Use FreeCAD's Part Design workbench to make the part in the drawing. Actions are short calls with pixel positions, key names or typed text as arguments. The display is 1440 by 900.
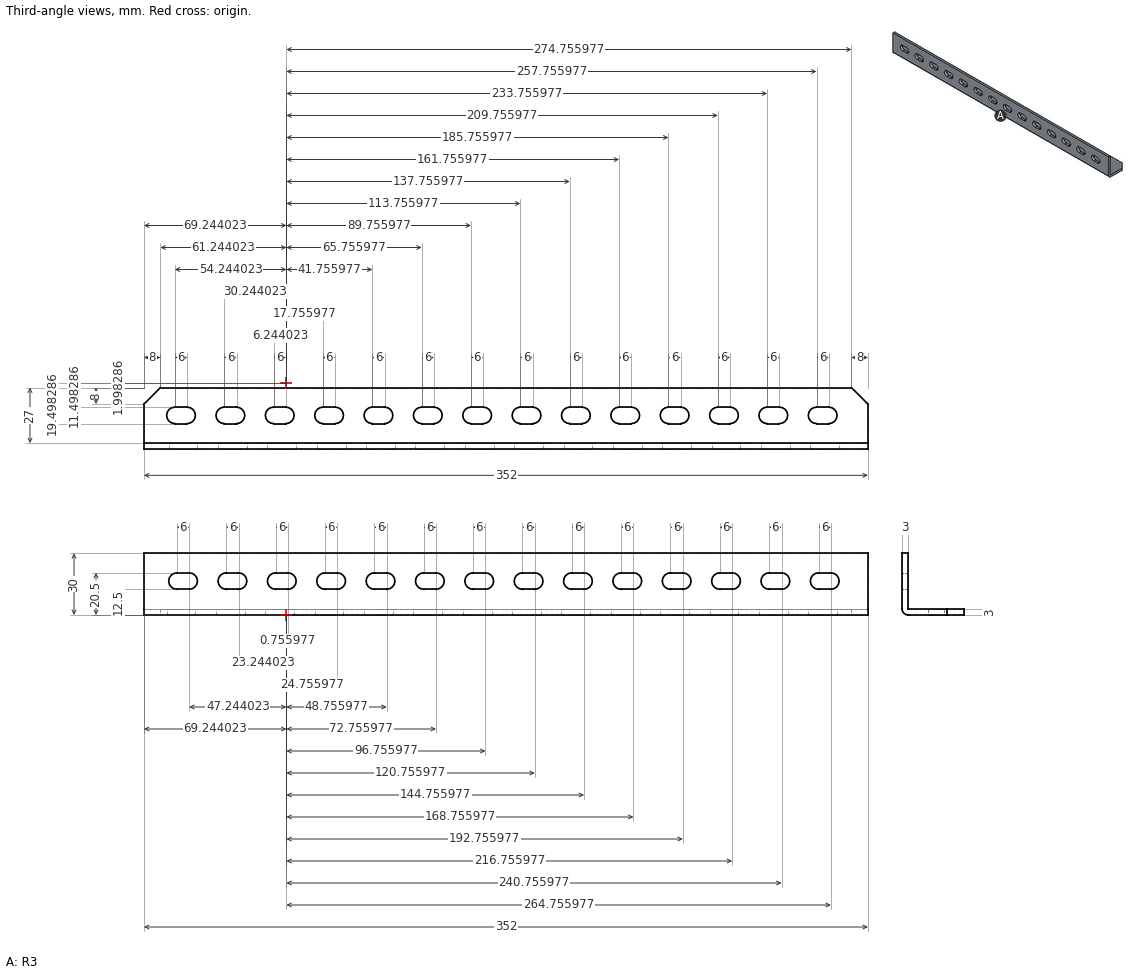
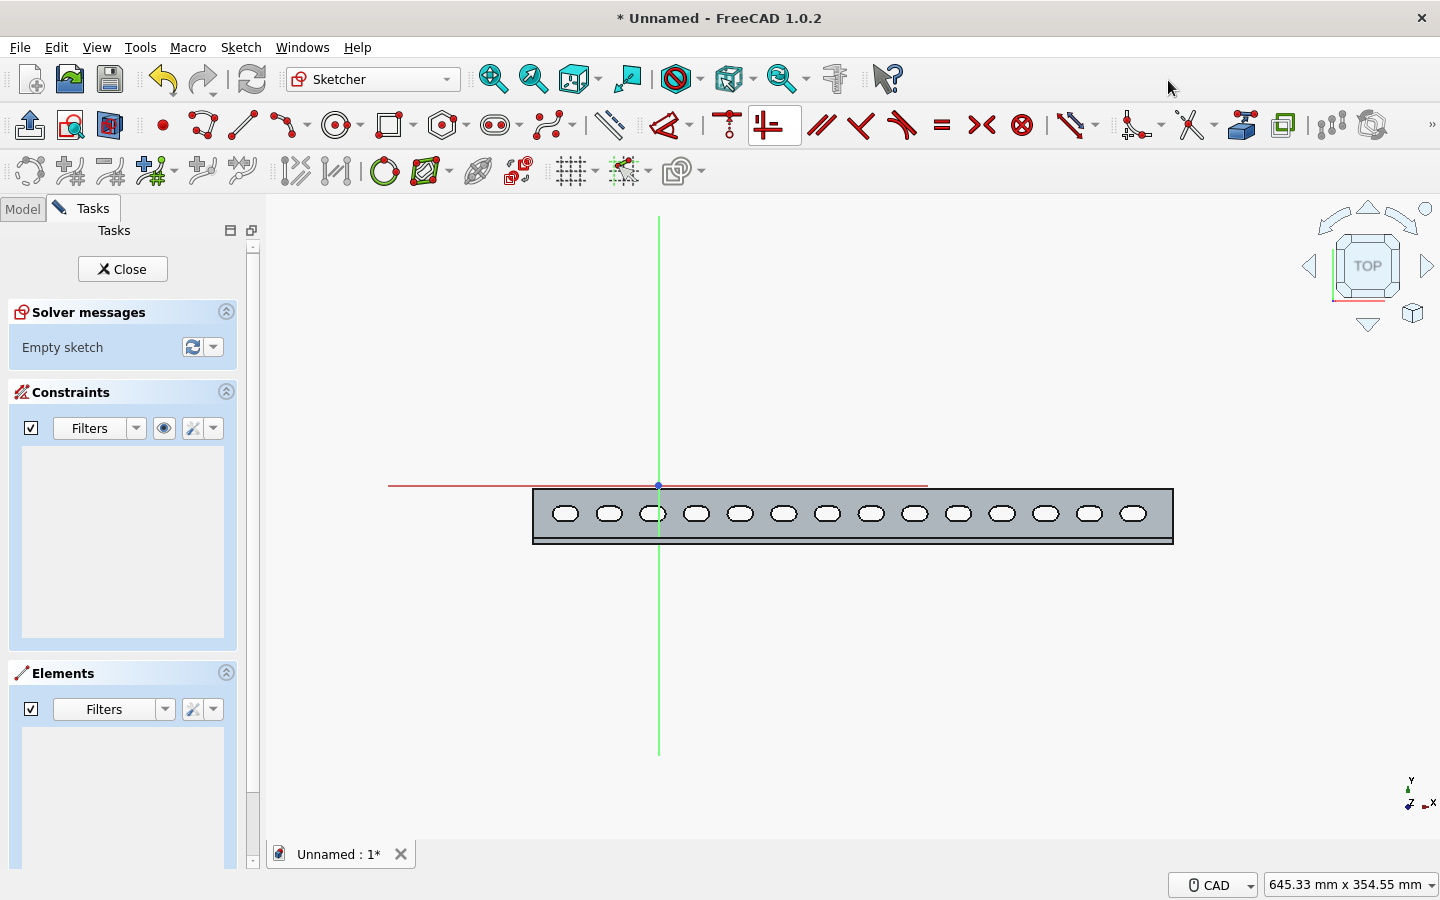
click(204, 126)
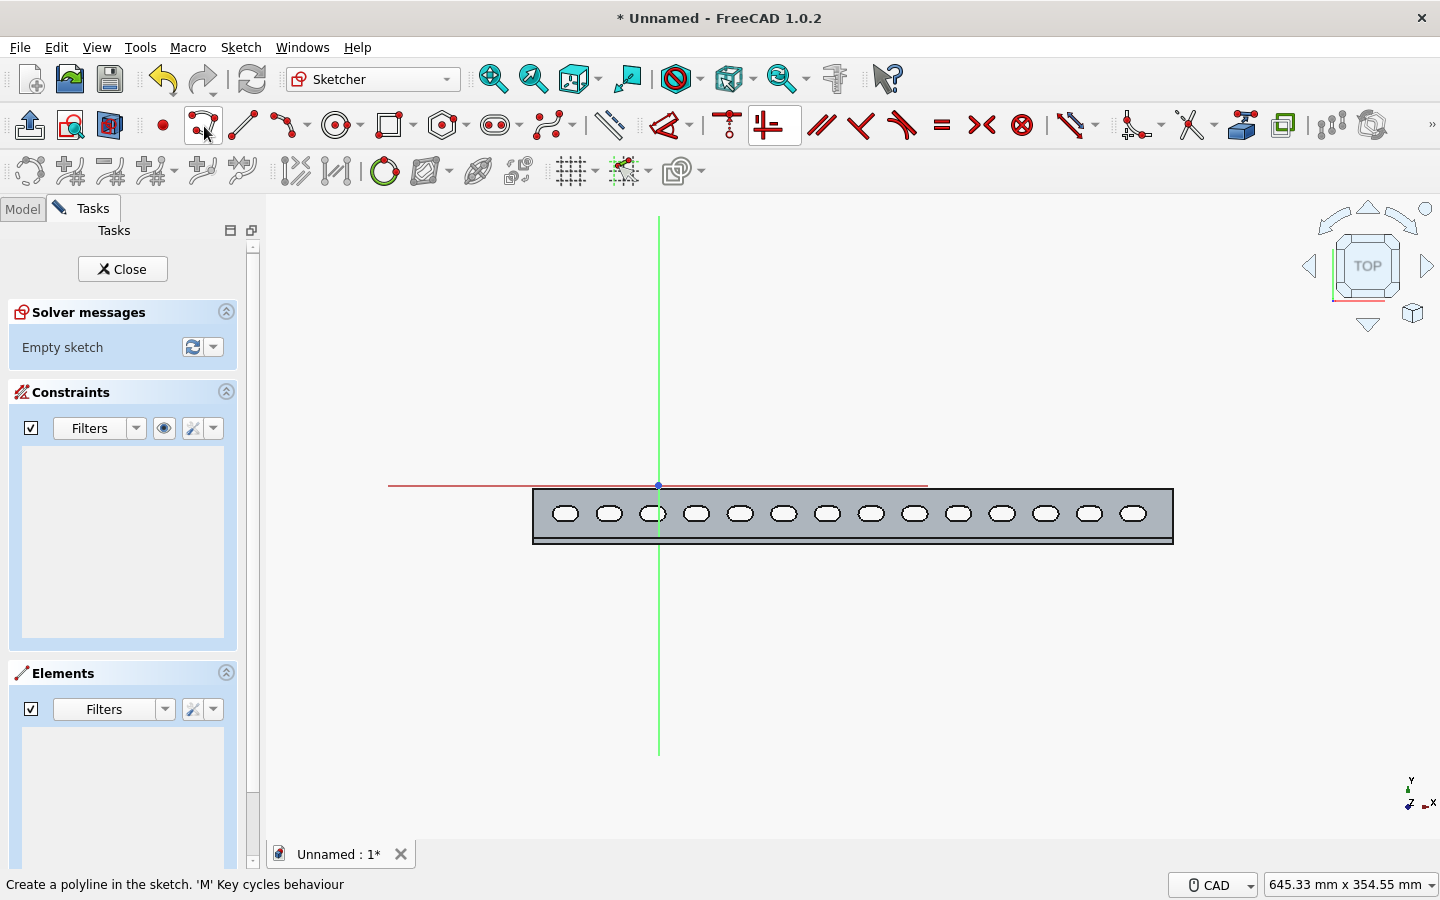
scroll(547, 489, up, 8)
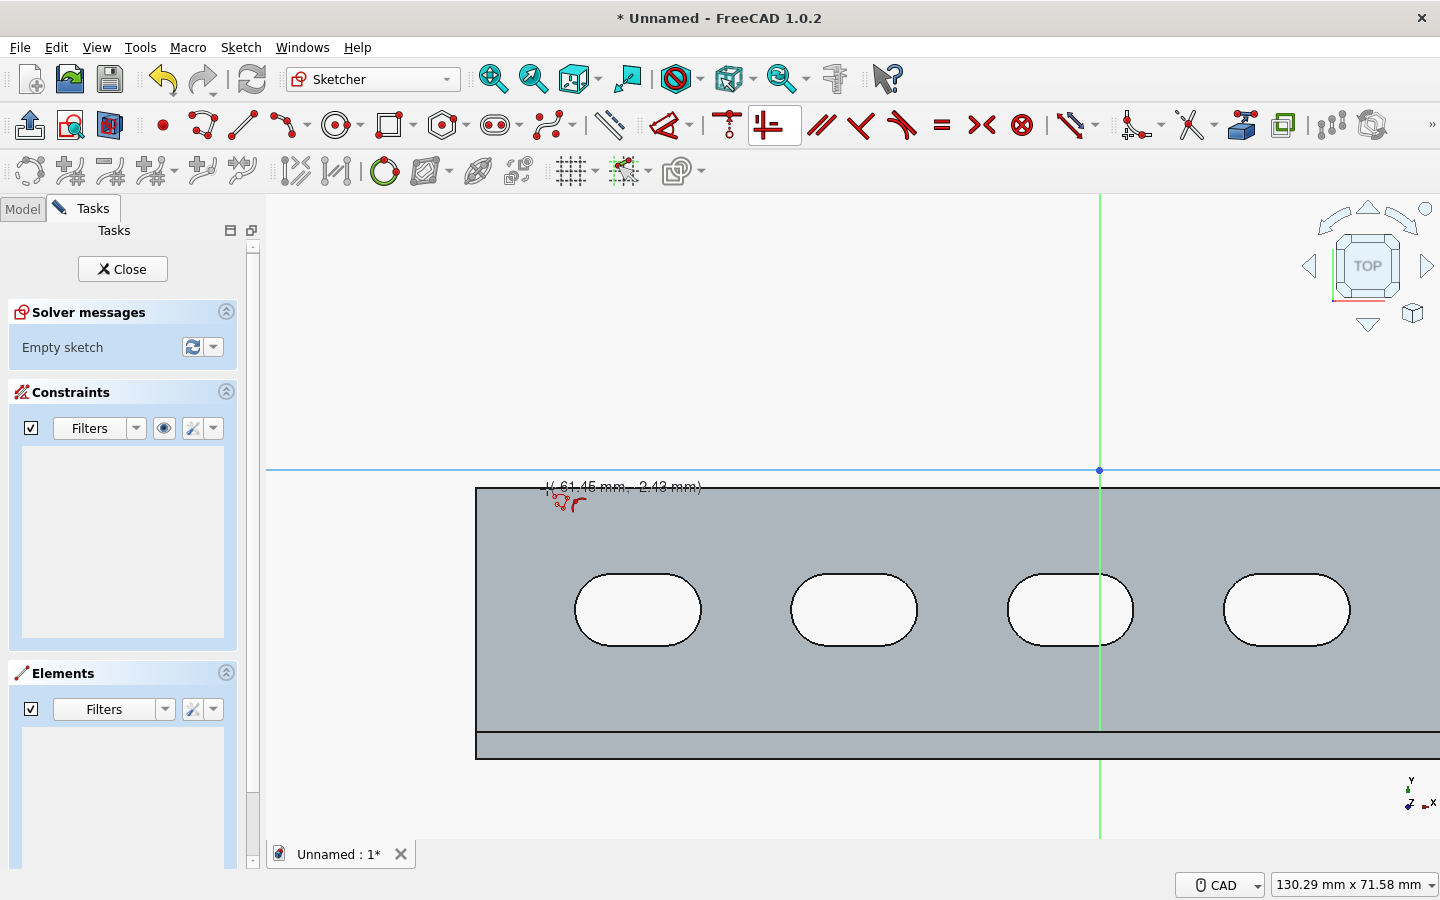
click(548, 488)
click(476, 488)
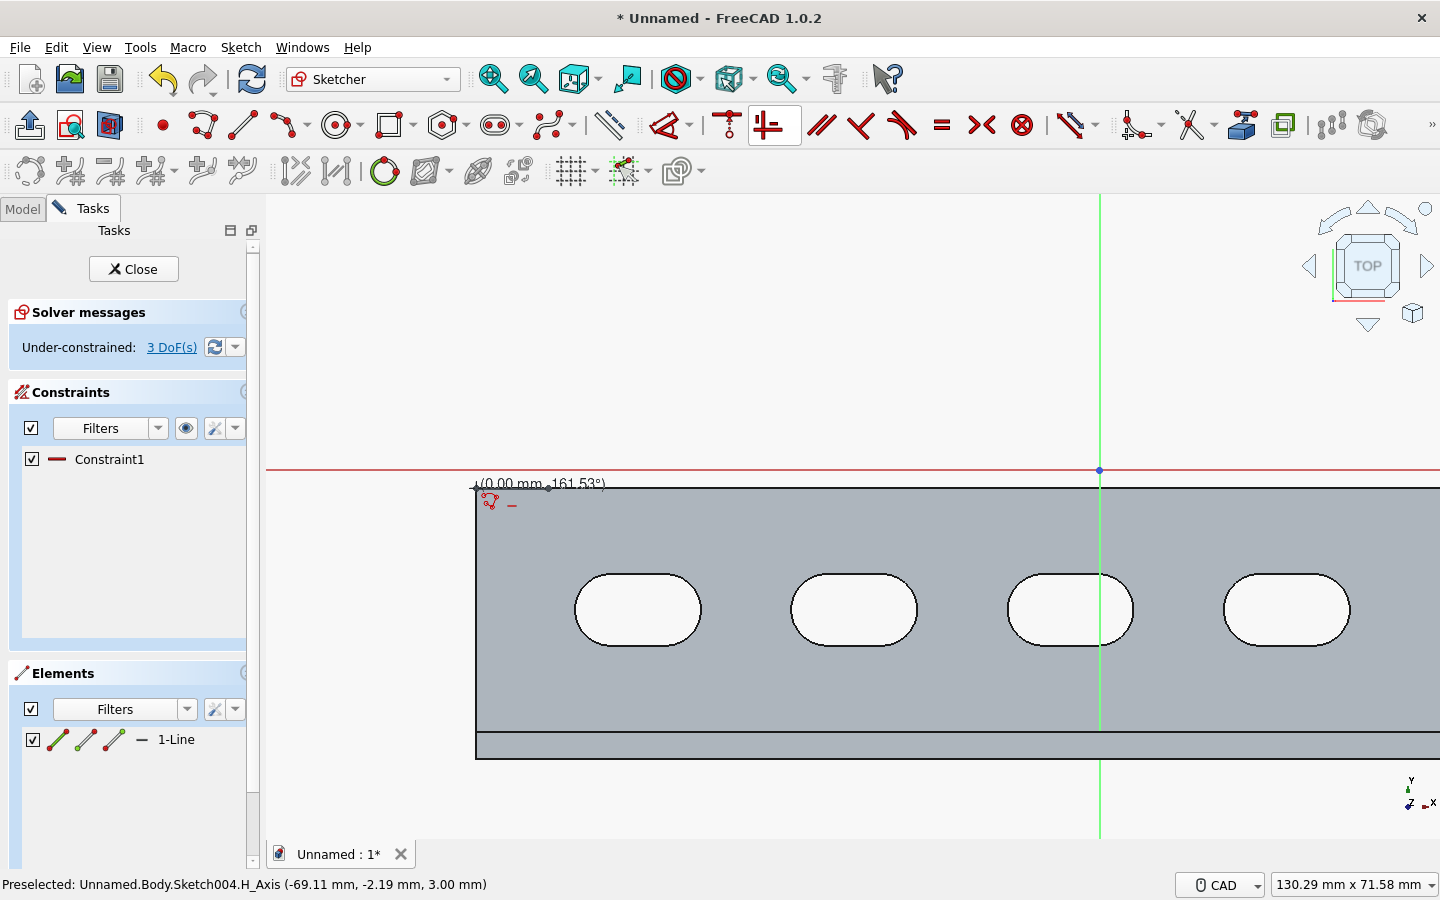
scroll(461, 517, down, 8)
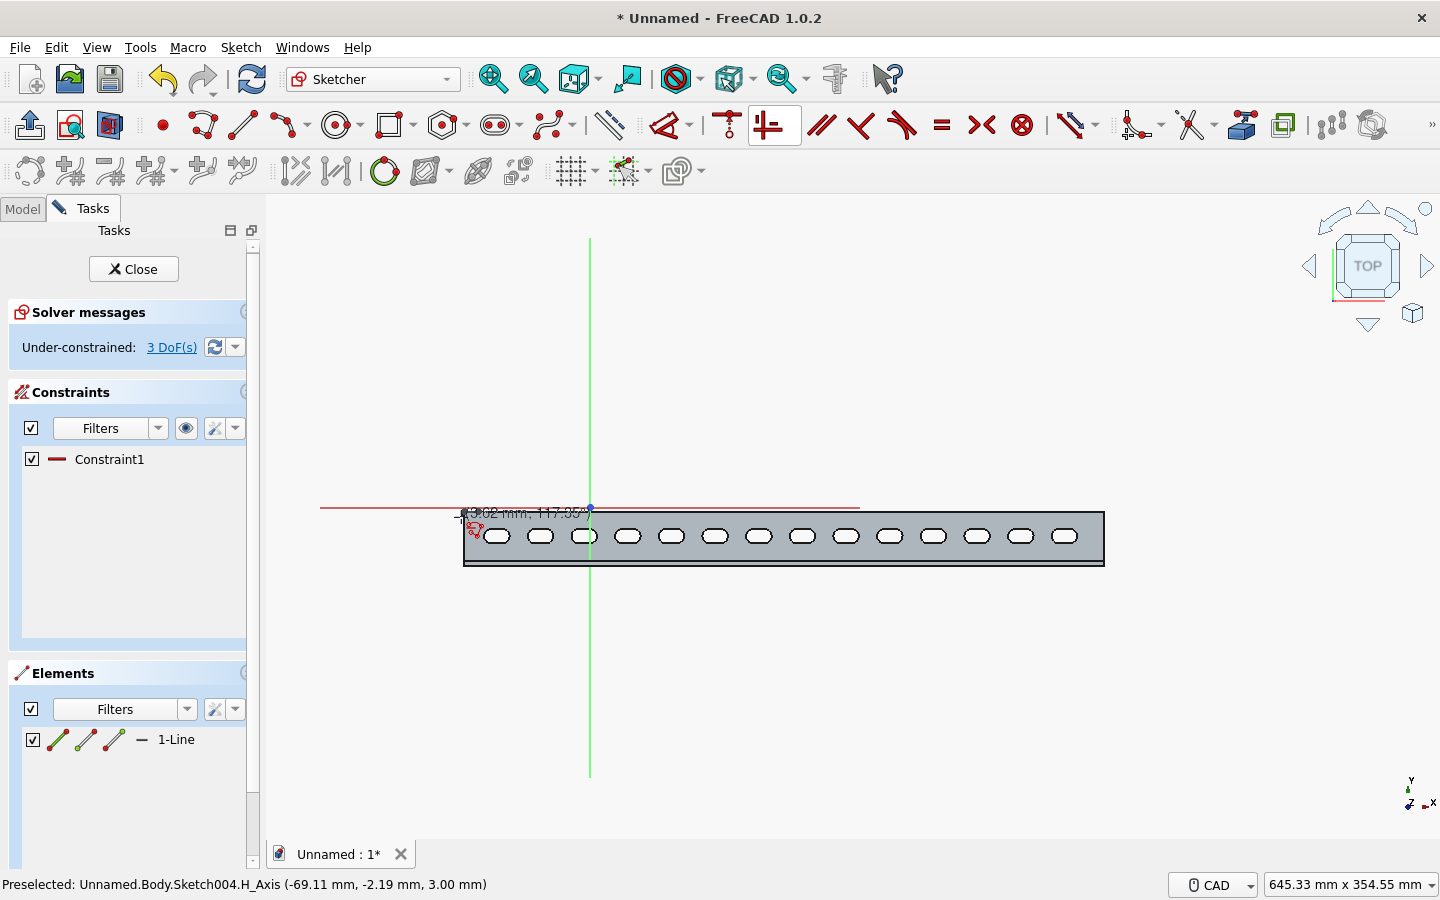
click(464, 526)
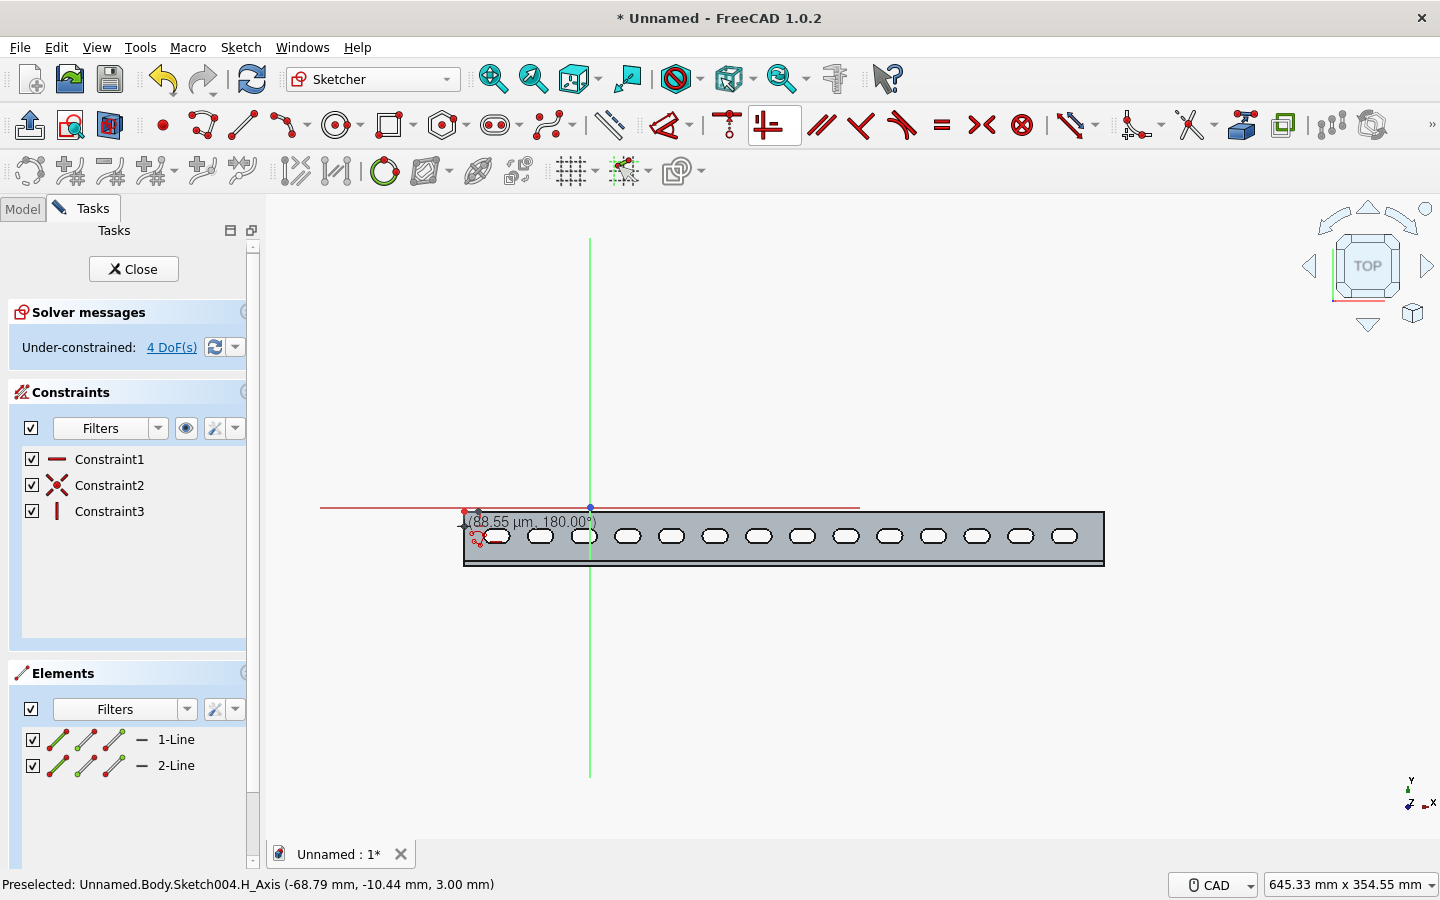
scroll(479, 512, up, 8)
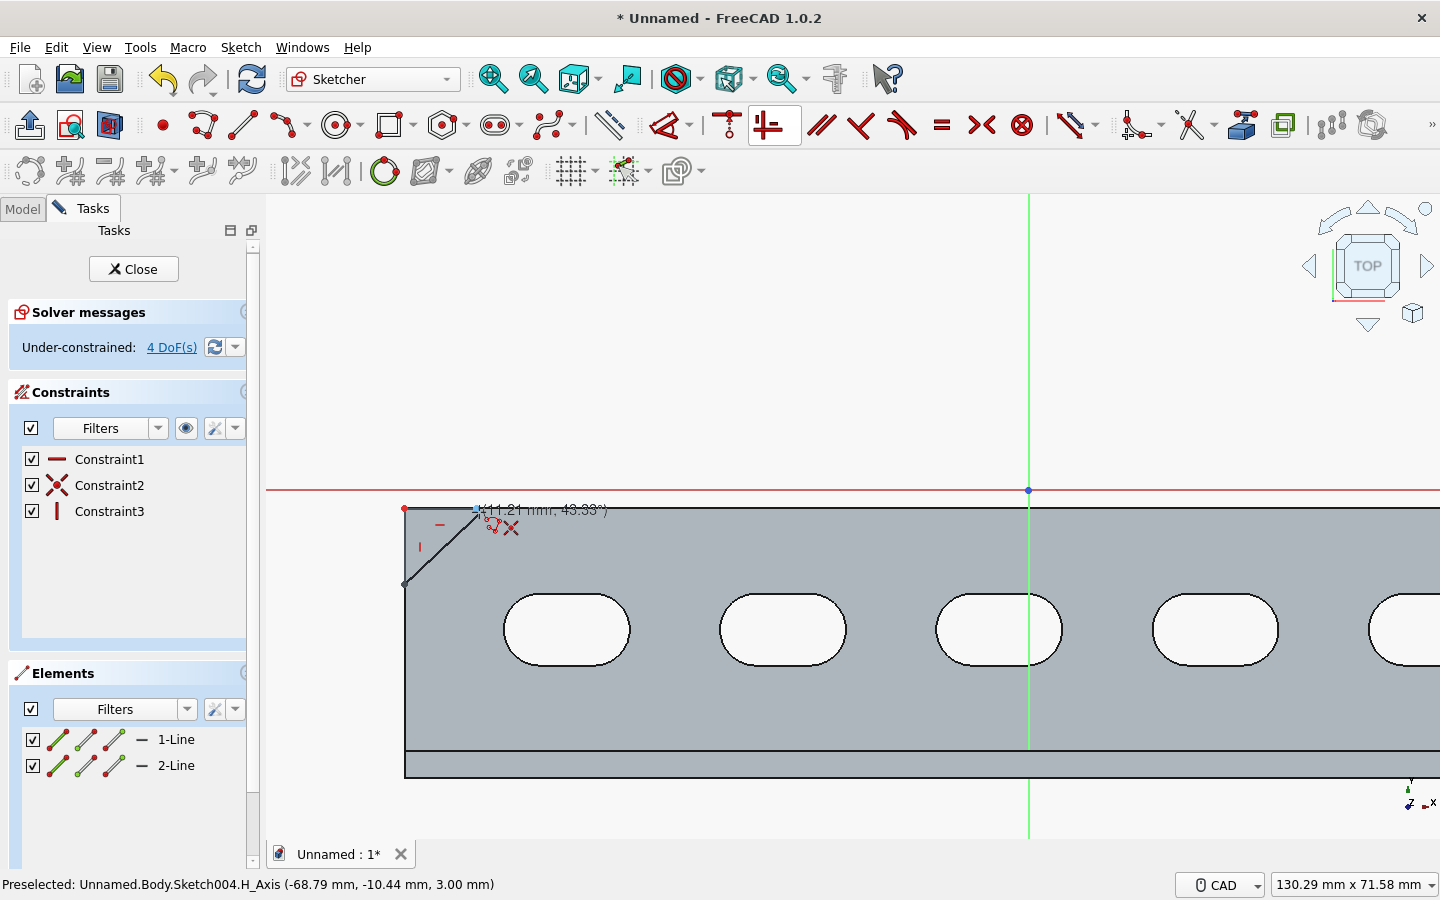
click(477, 509)